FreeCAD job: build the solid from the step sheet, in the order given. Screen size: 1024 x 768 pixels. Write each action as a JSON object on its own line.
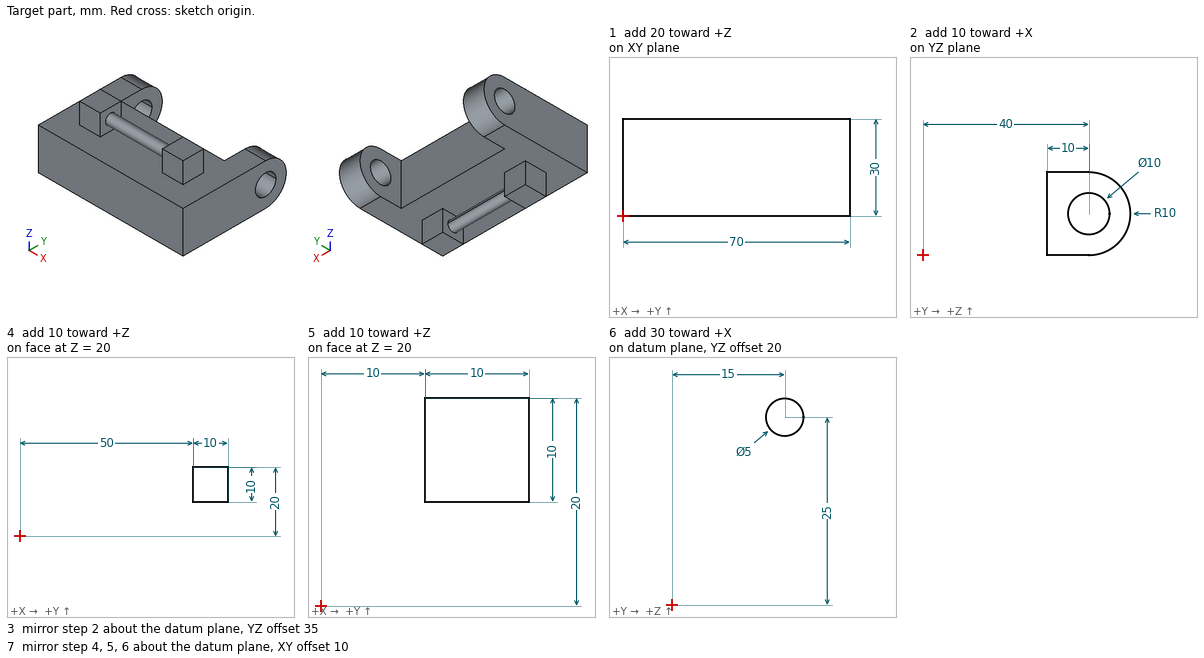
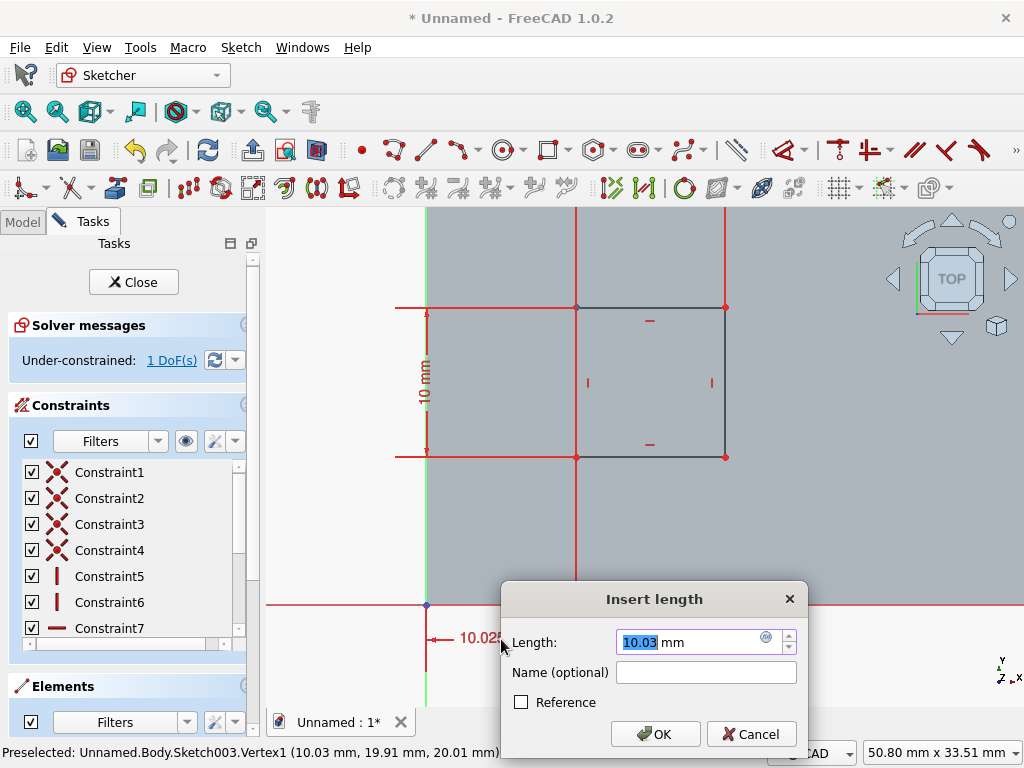
{"action": "type", "text": "10"}
{"action": "key", "text": "Return"}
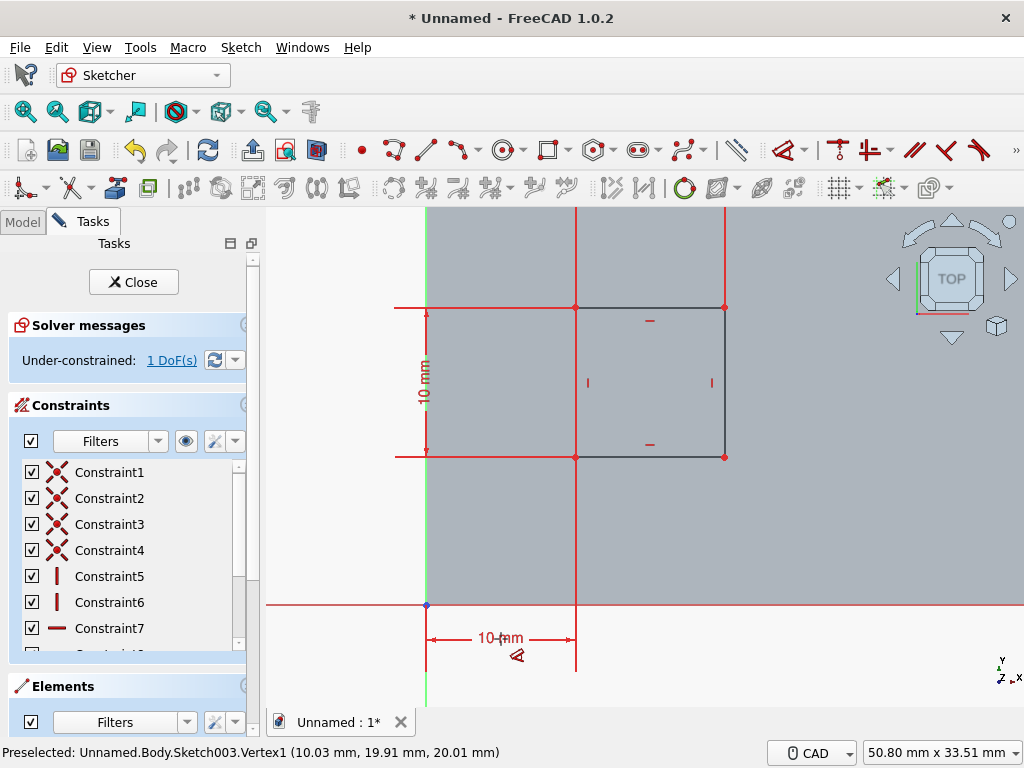
{"action": "left_click", "coordinate": [576, 308]}
{"action": "left_click", "coordinate": [392, 457]}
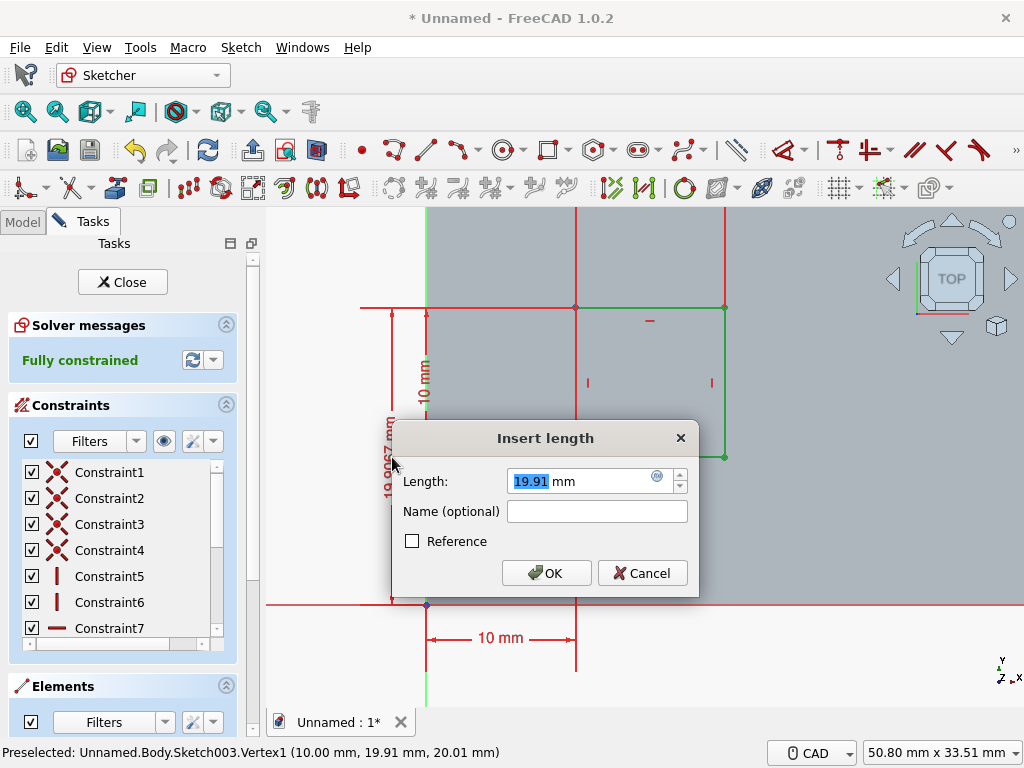
{"action": "type", "text": "20"}
{"action": "key", "text": "Return"}
{"action": "key", "text": "Escape"}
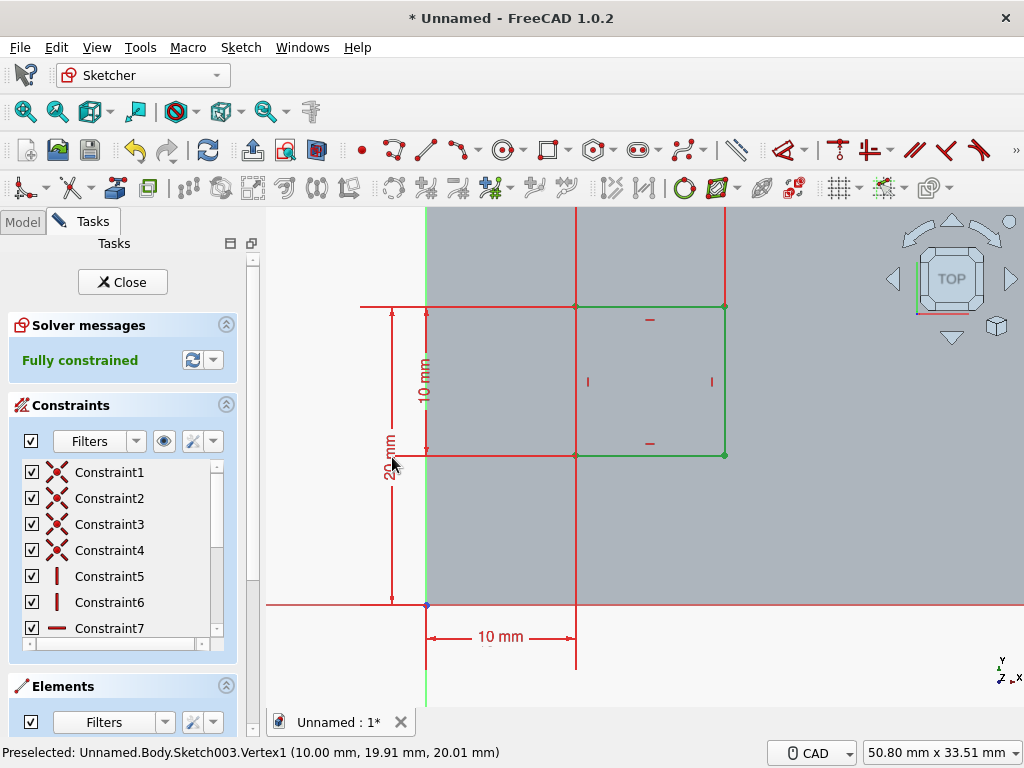
{"action": "left_click", "coordinate": [123, 282]}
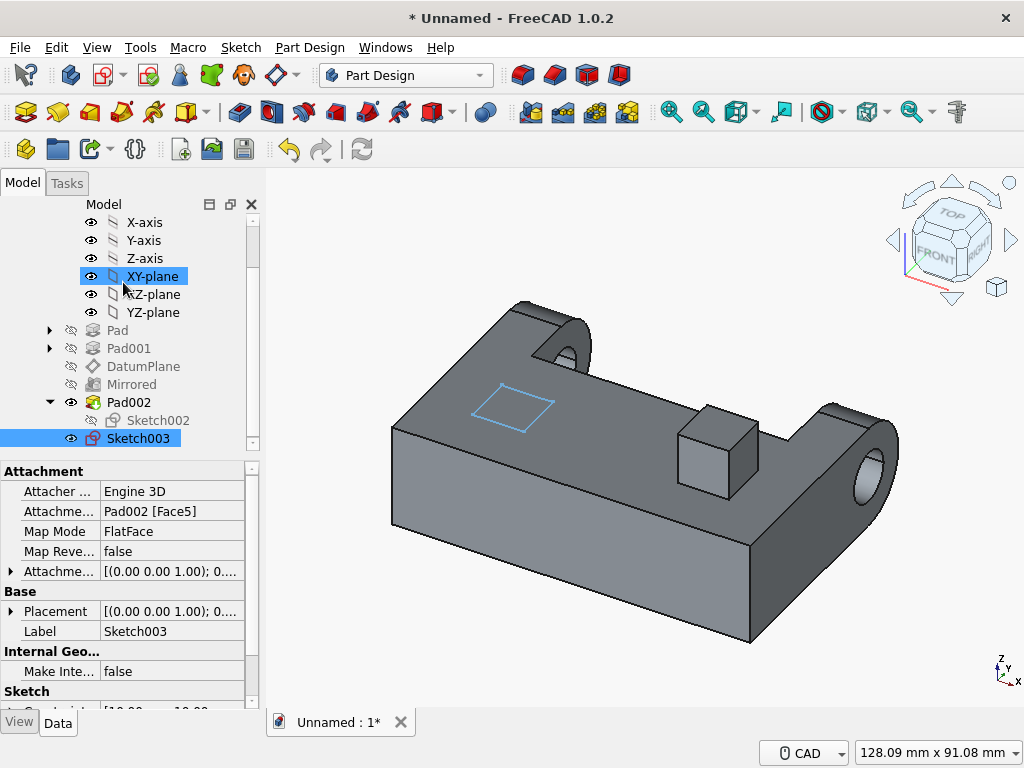
{"action": "left_click", "coordinate": [26, 112]}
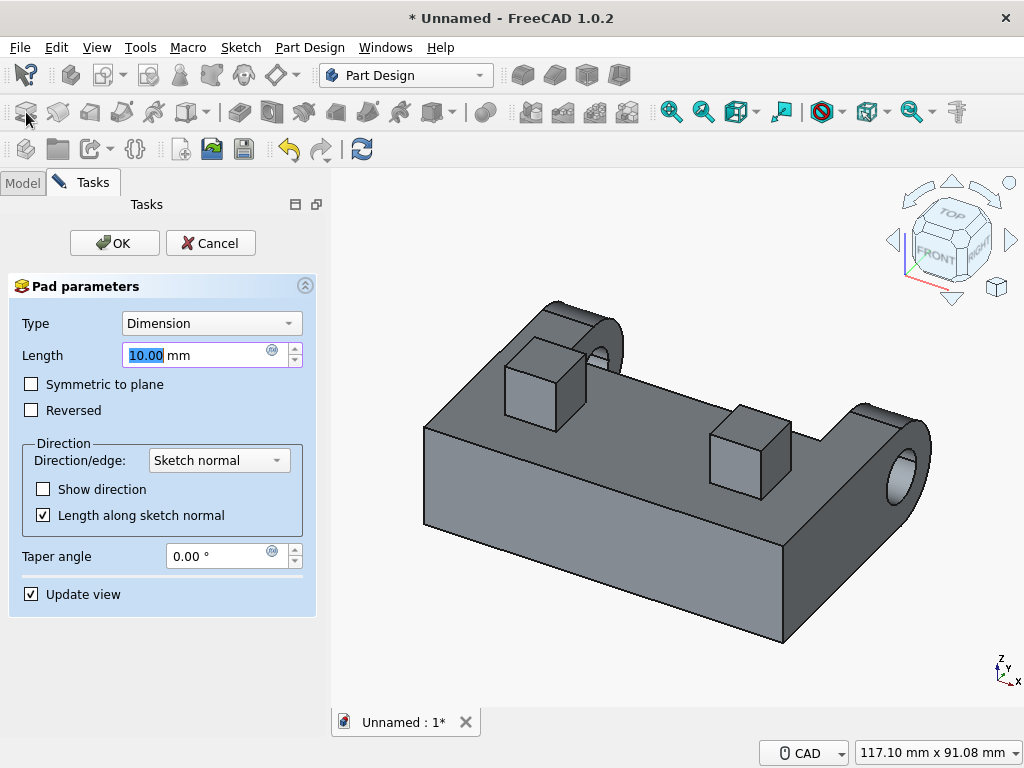
{"action": "type", "text": "10"}
{"action": "key", "text": "Tab"}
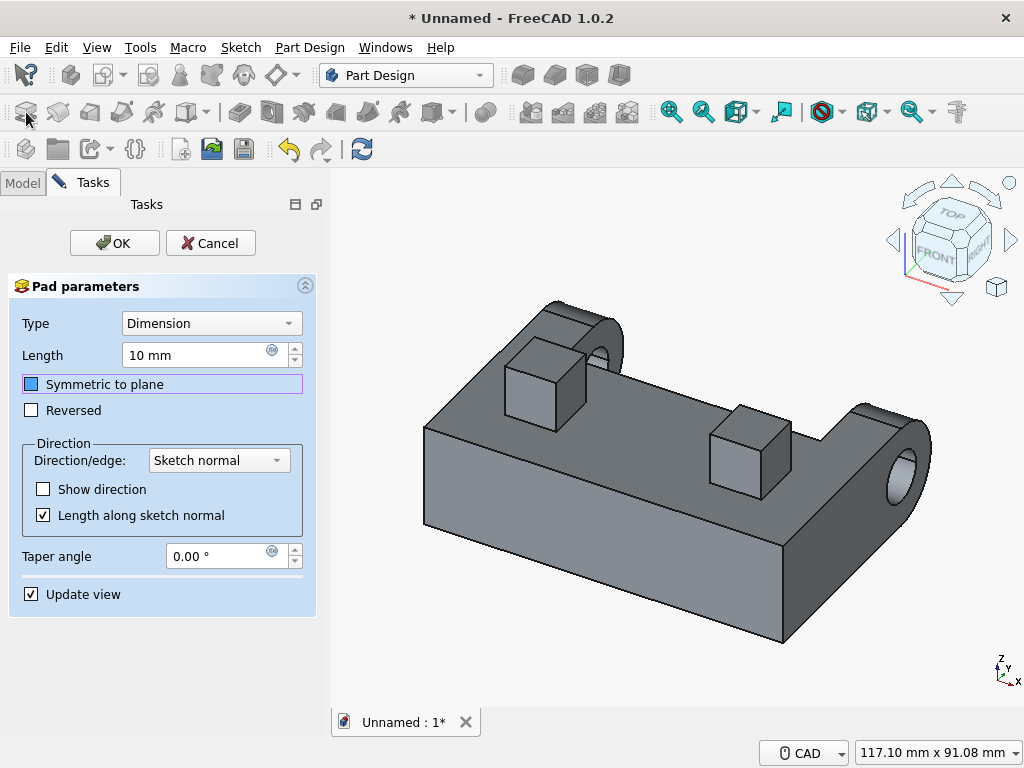
{"action": "left_click", "coordinate": [115, 243]}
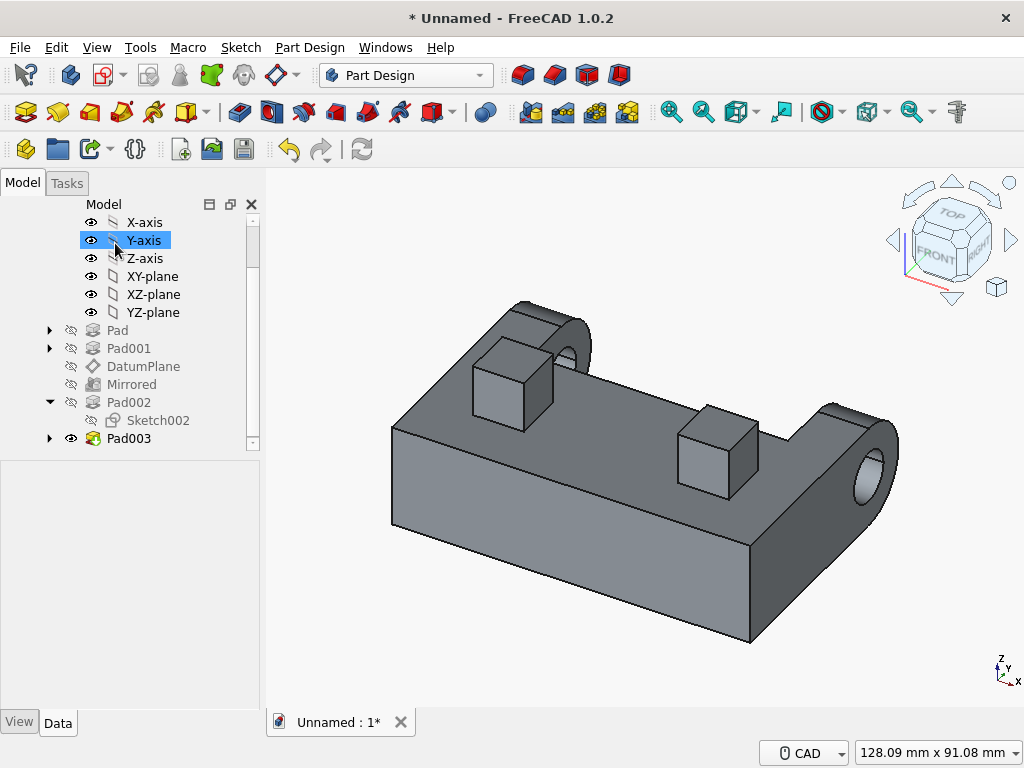
{"action": "scroll", "coordinate": [160, 326], "scroll_direction": "down", "scroll_amount": 3}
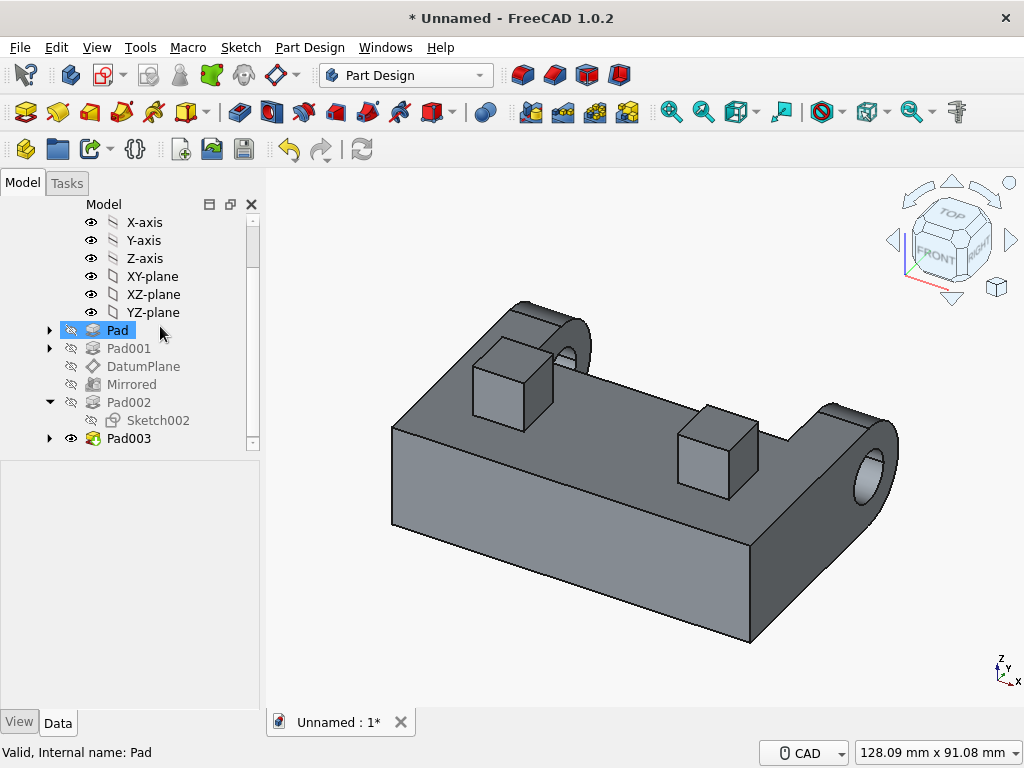
{"action": "scroll", "coordinate": [160, 326], "scroll_direction": "up", "scroll_amount": 15}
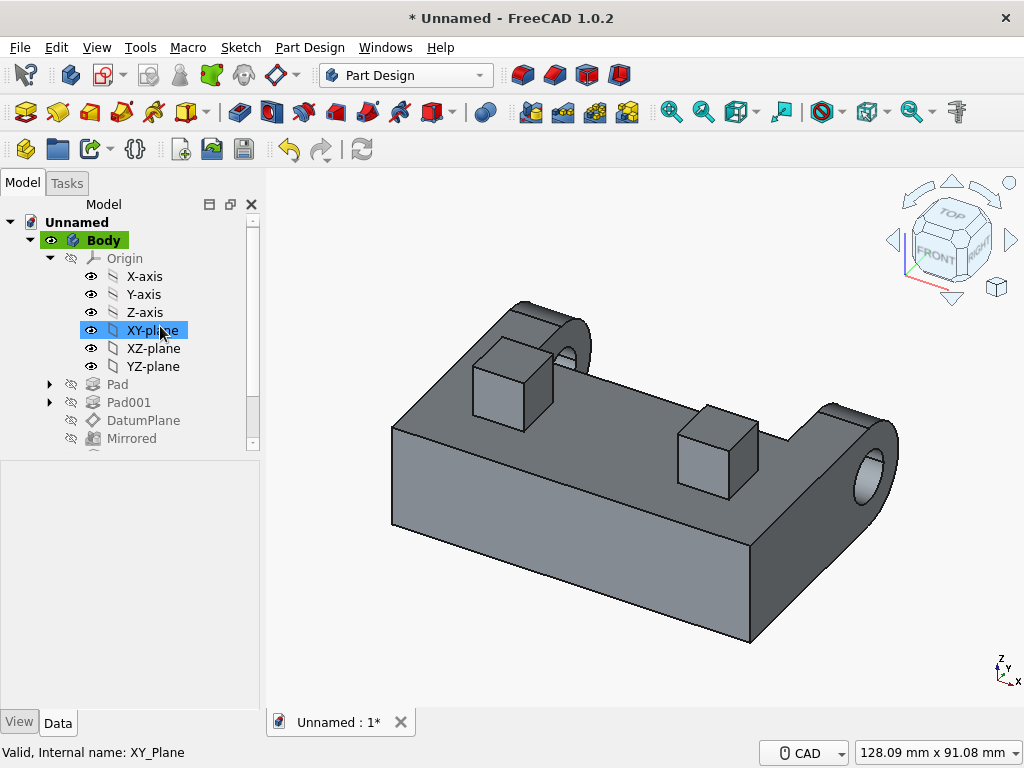
{"action": "left_click", "coordinate": [136, 366]}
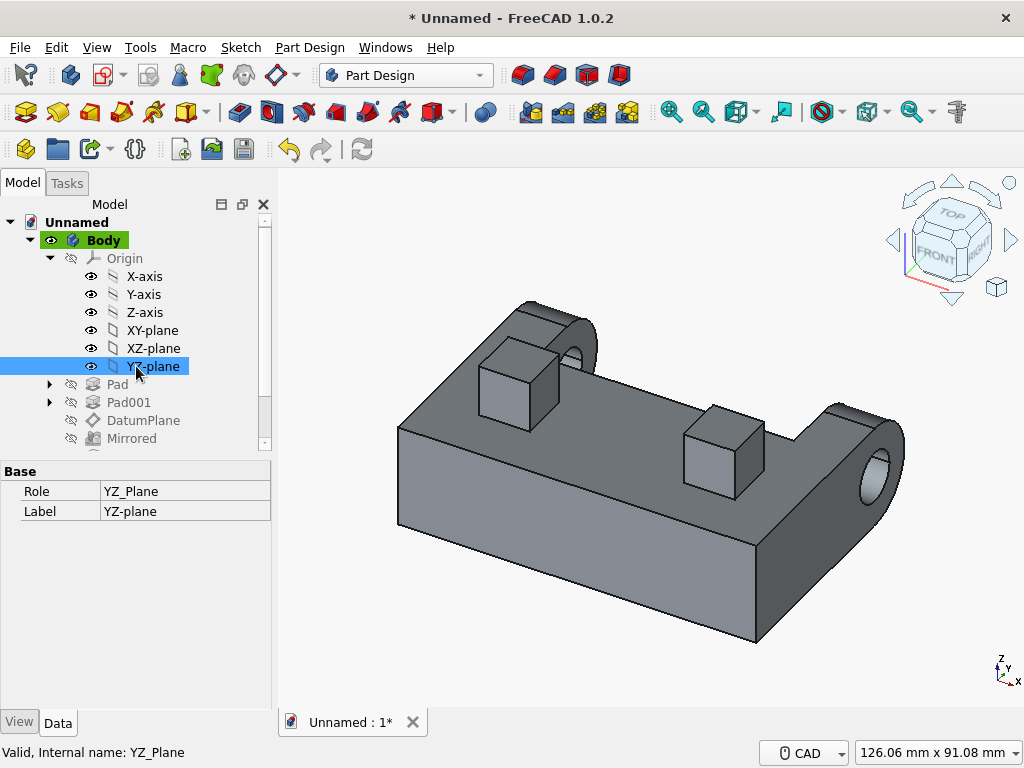
{"action": "left_click", "coordinate": [276, 76]}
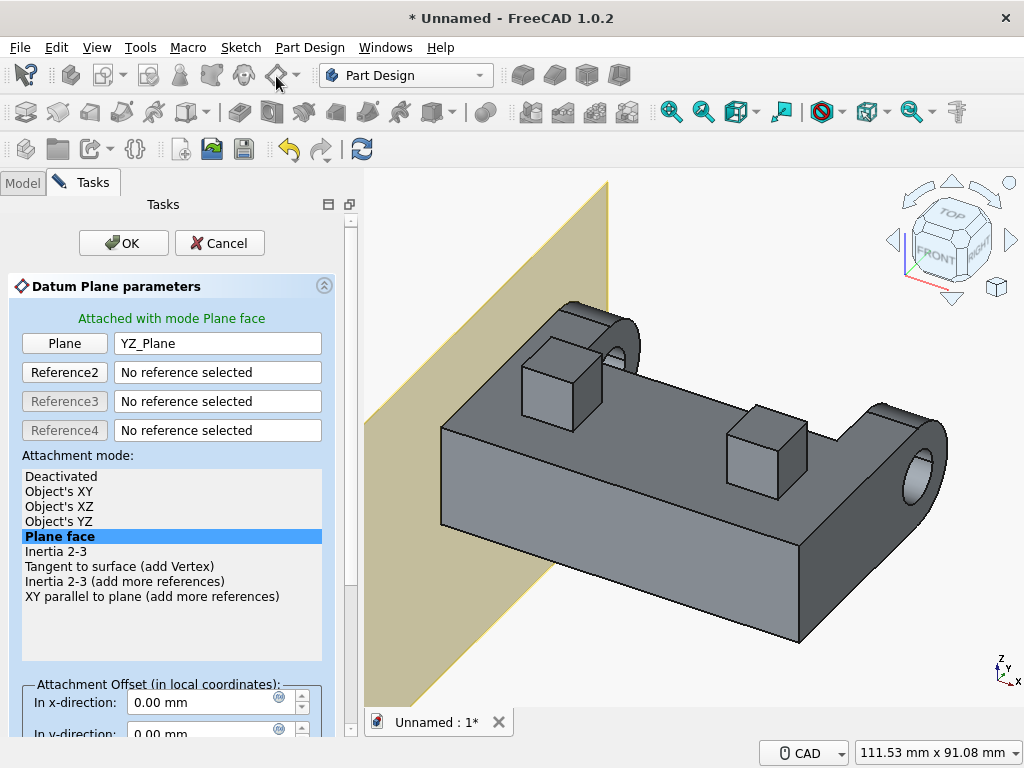
{"action": "scroll", "coordinate": [351, 475], "scroll_direction": "down", "scroll_amount": 2}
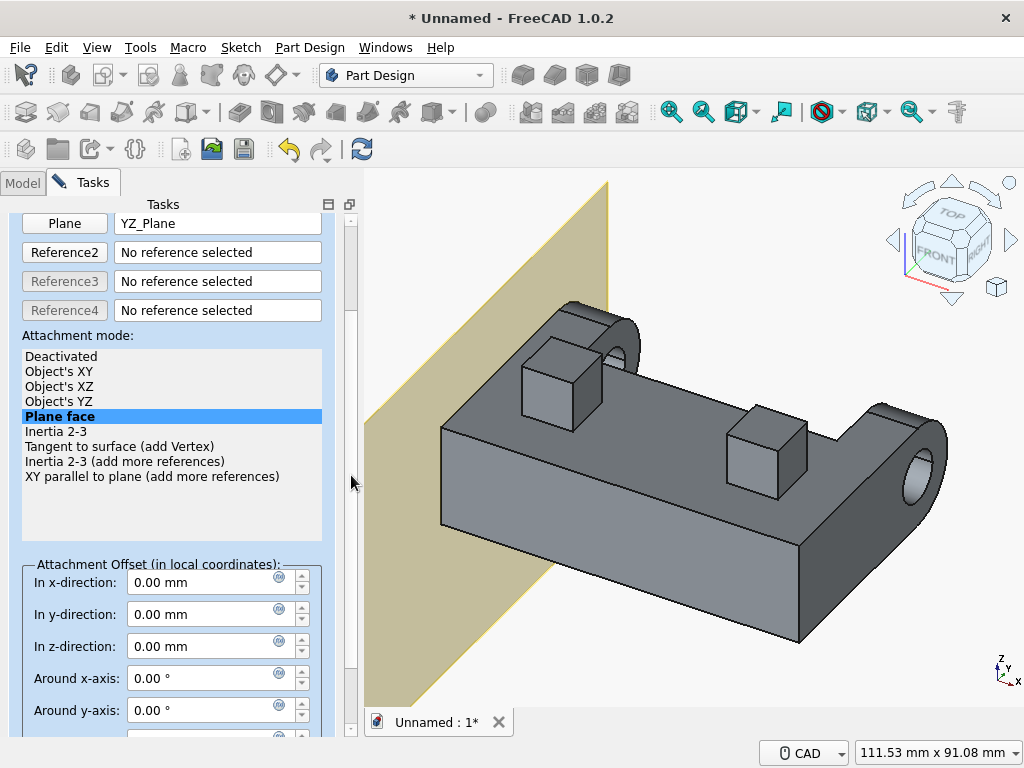
{"action": "triple_click", "coordinate": [210, 646]}